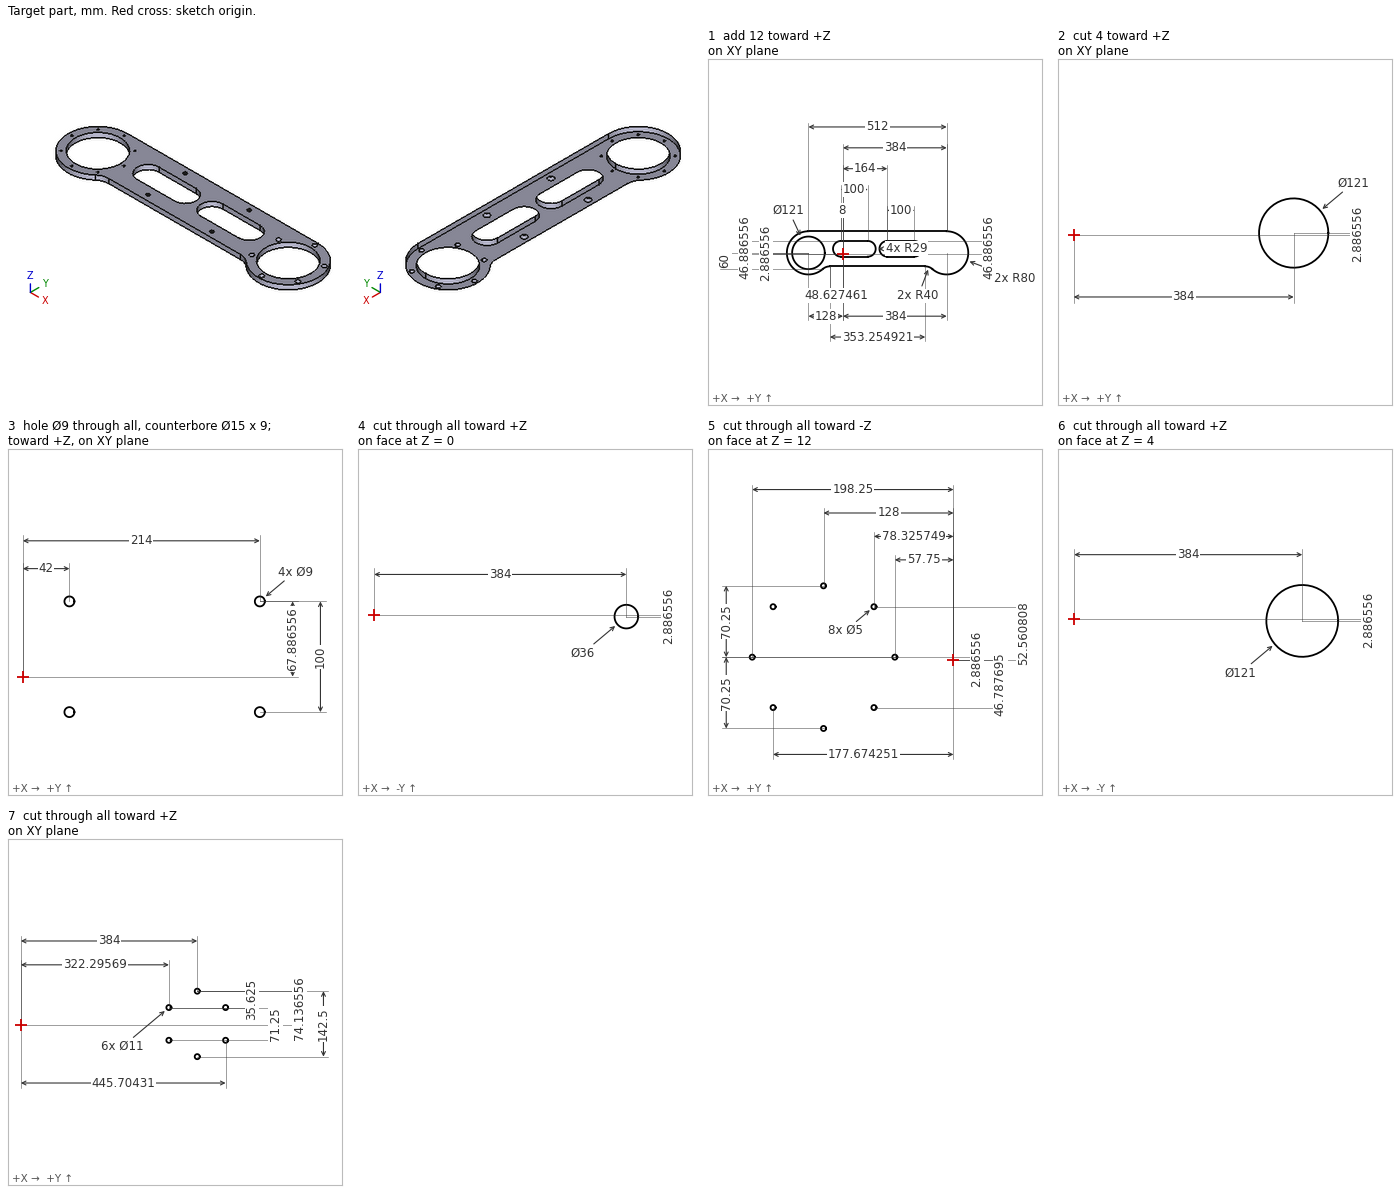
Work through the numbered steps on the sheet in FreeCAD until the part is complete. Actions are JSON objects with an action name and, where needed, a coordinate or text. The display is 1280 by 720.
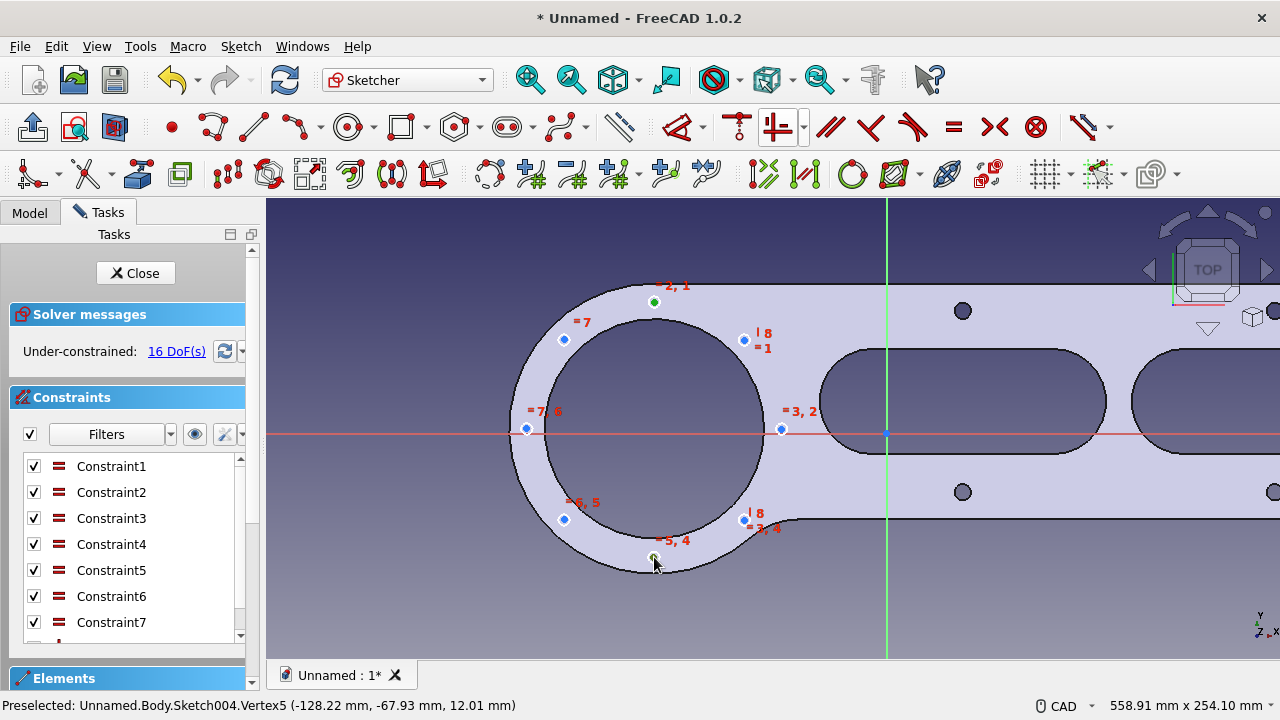
{"action": "left_click", "coordinate": [804, 128]}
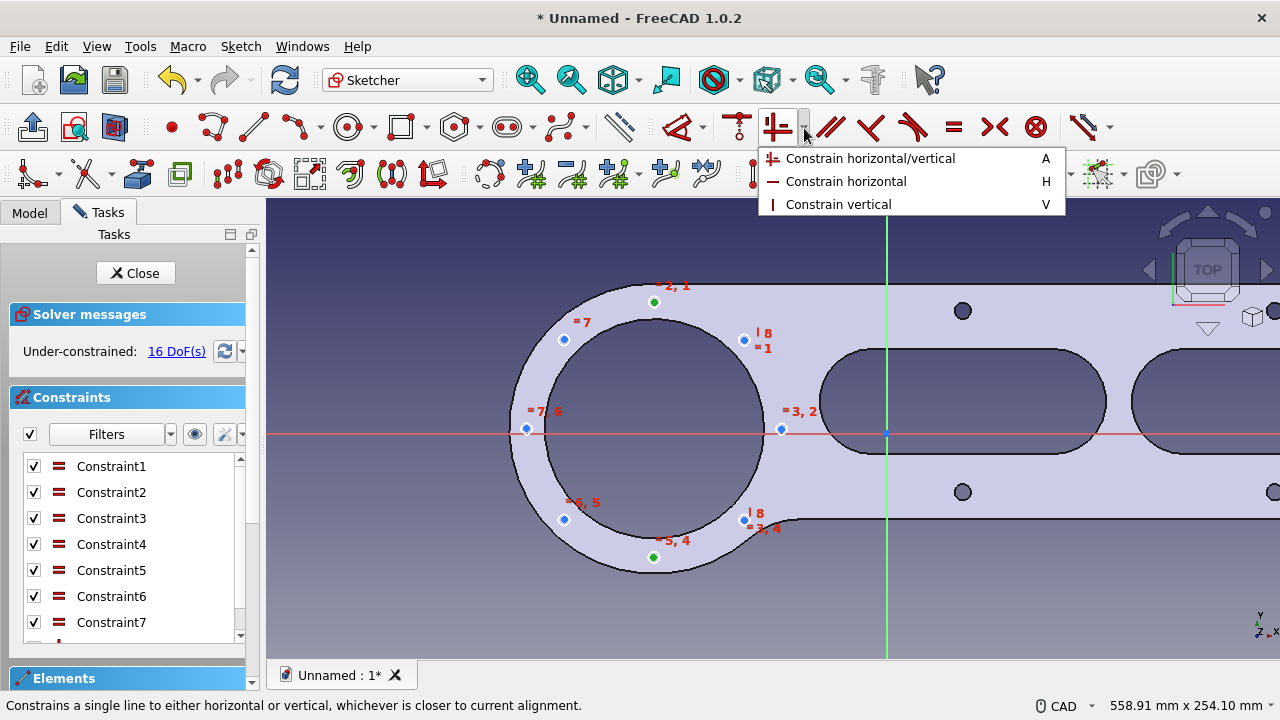
{"action": "left_click", "coordinate": [912, 204]}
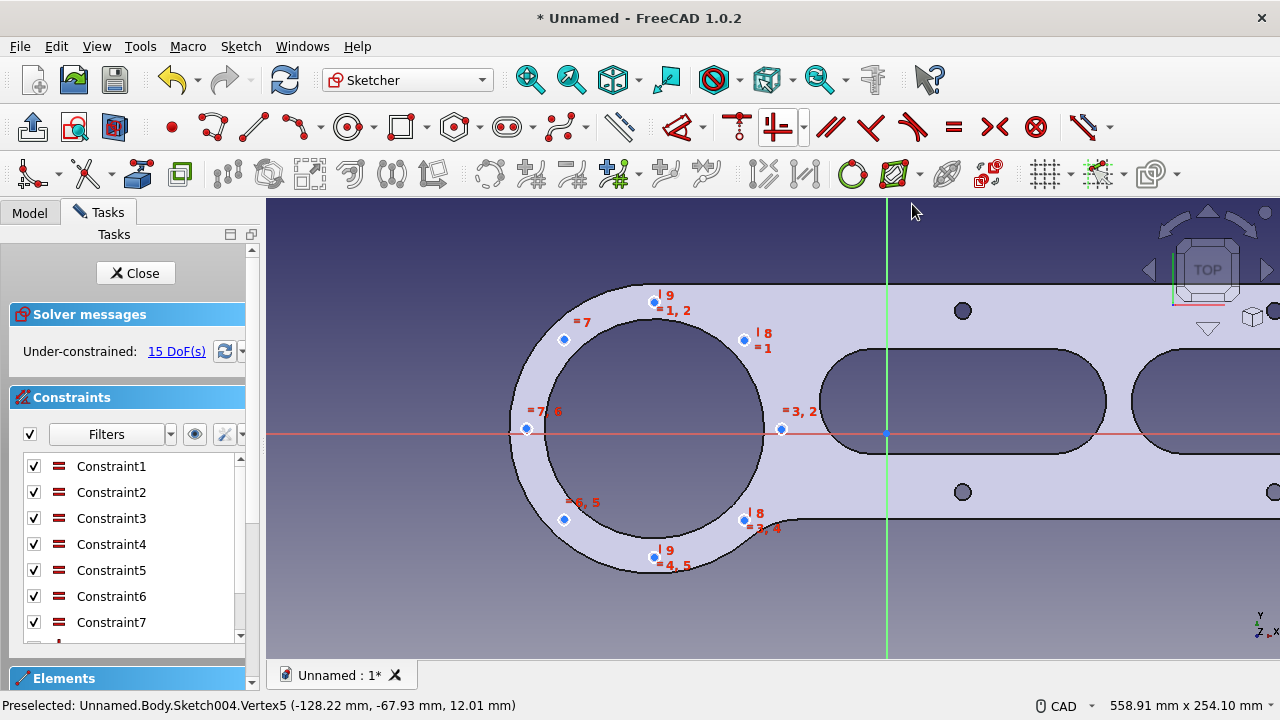
{"action": "left_click", "coordinate": [744, 520]}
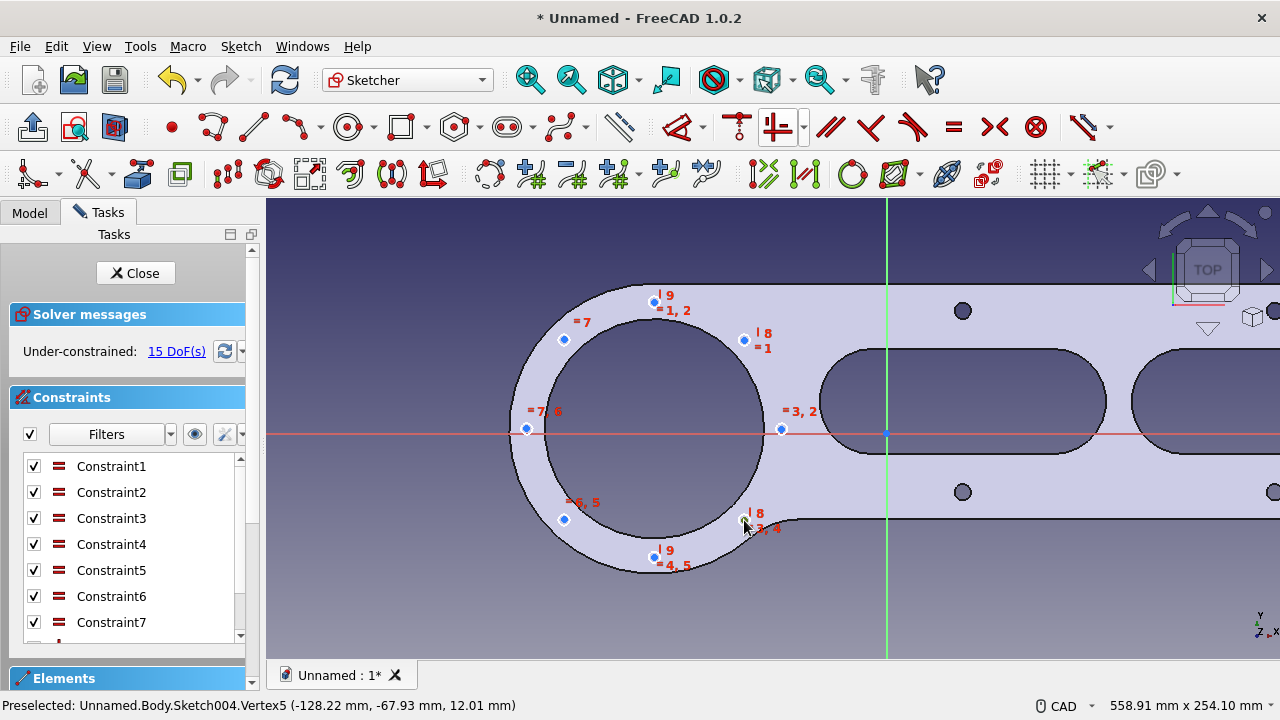
{"action": "left_click", "coordinate": [564, 520]}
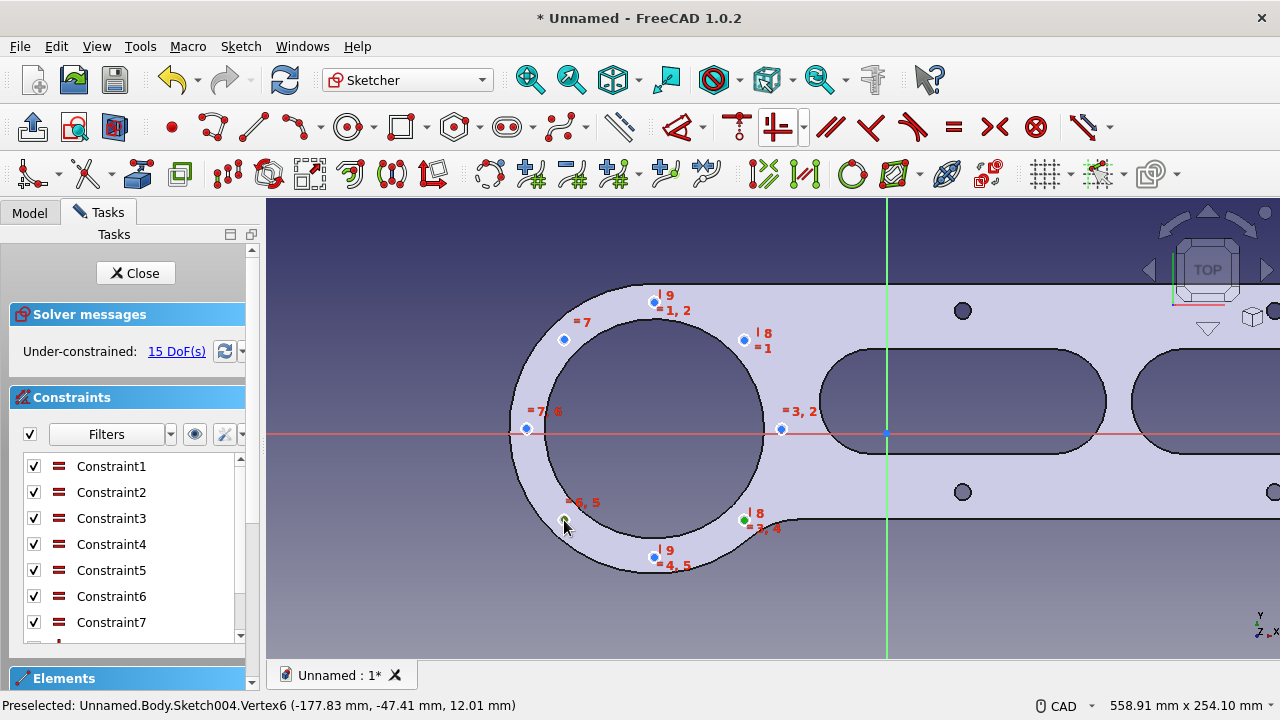
{"action": "left_click", "coordinate": [804, 128]}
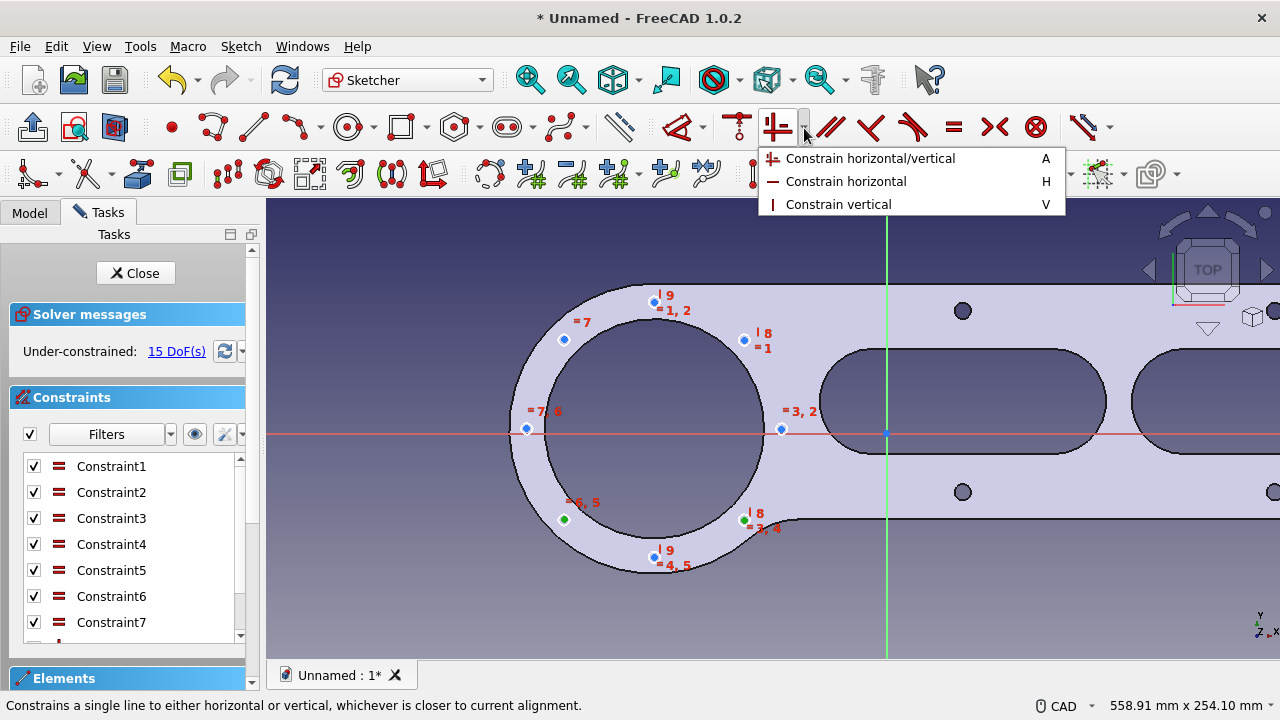
{"action": "left_click", "coordinate": [912, 182]}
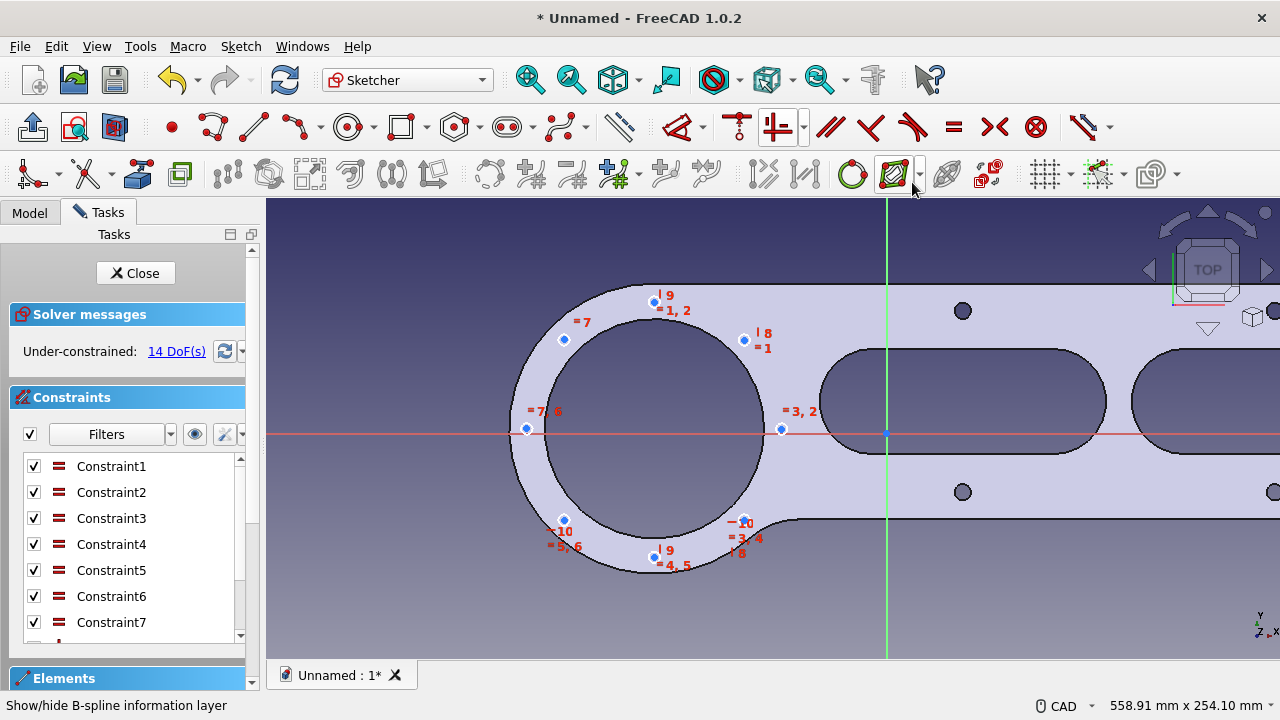
{"action": "left_click", "coordinate": [782, 429]}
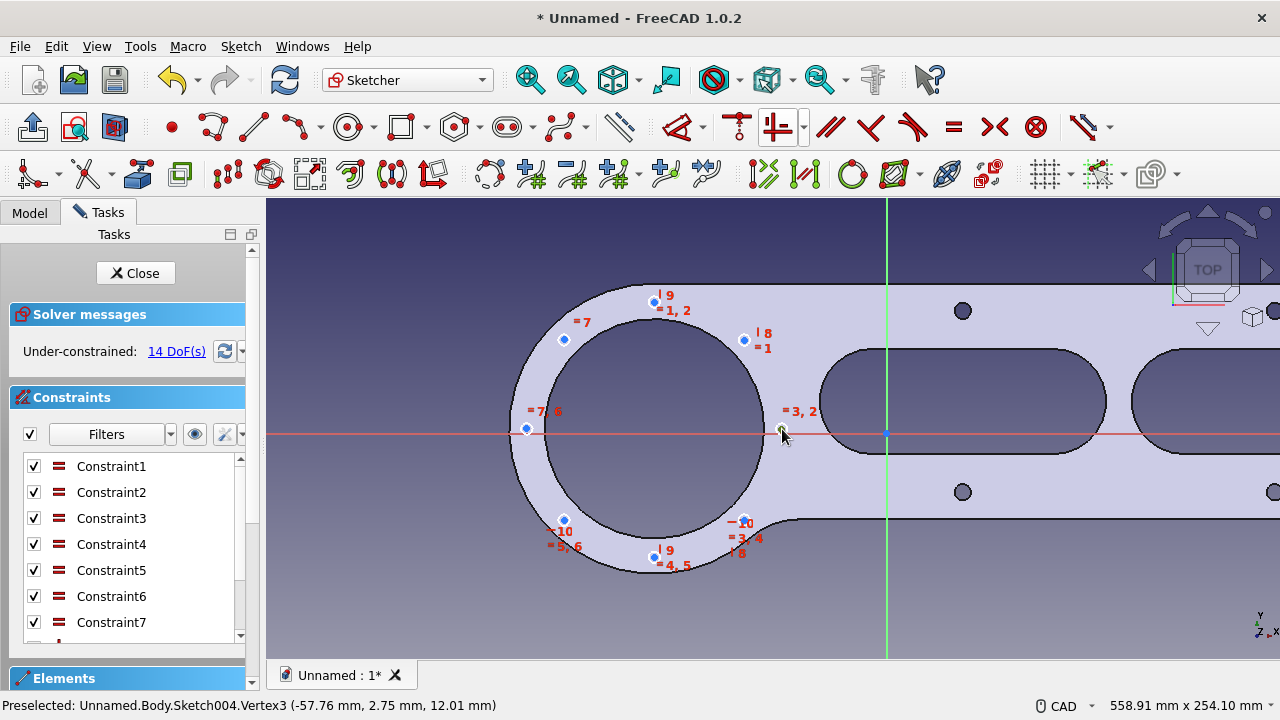
{"action": "left_click", "coordinate": [527, 429]}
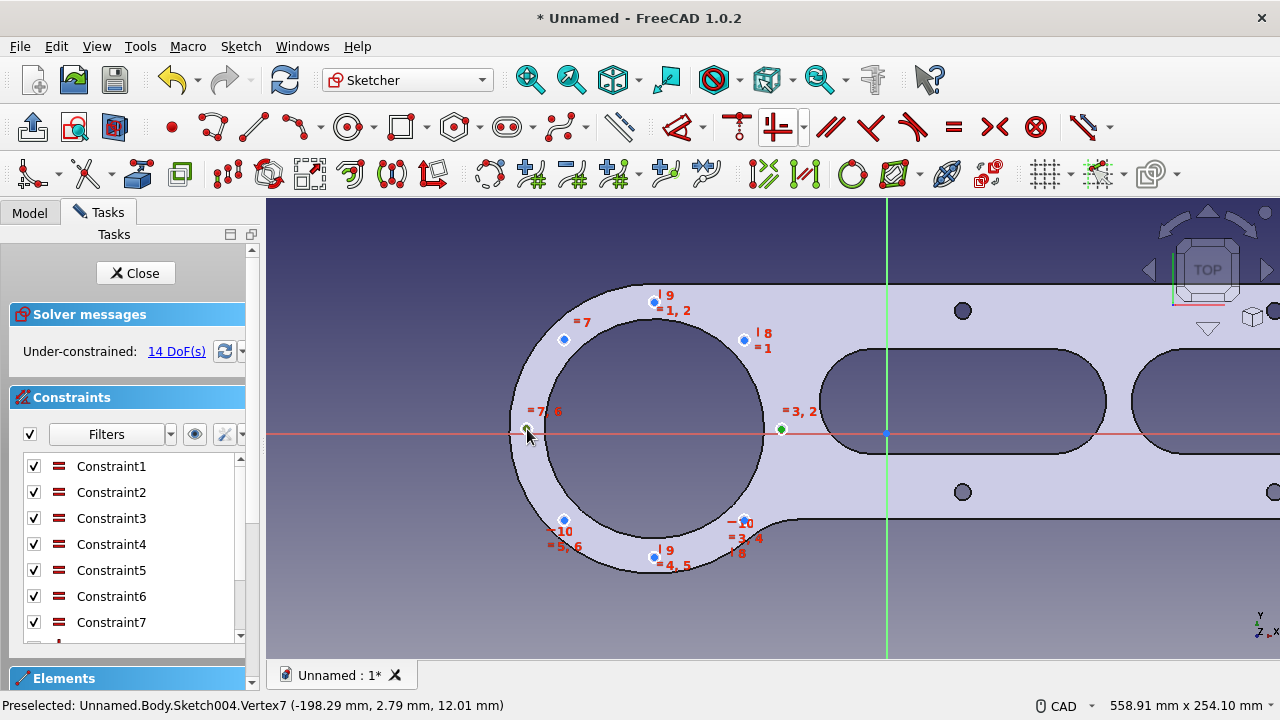
{"action": "left_click", "coordinate": [804, 128]}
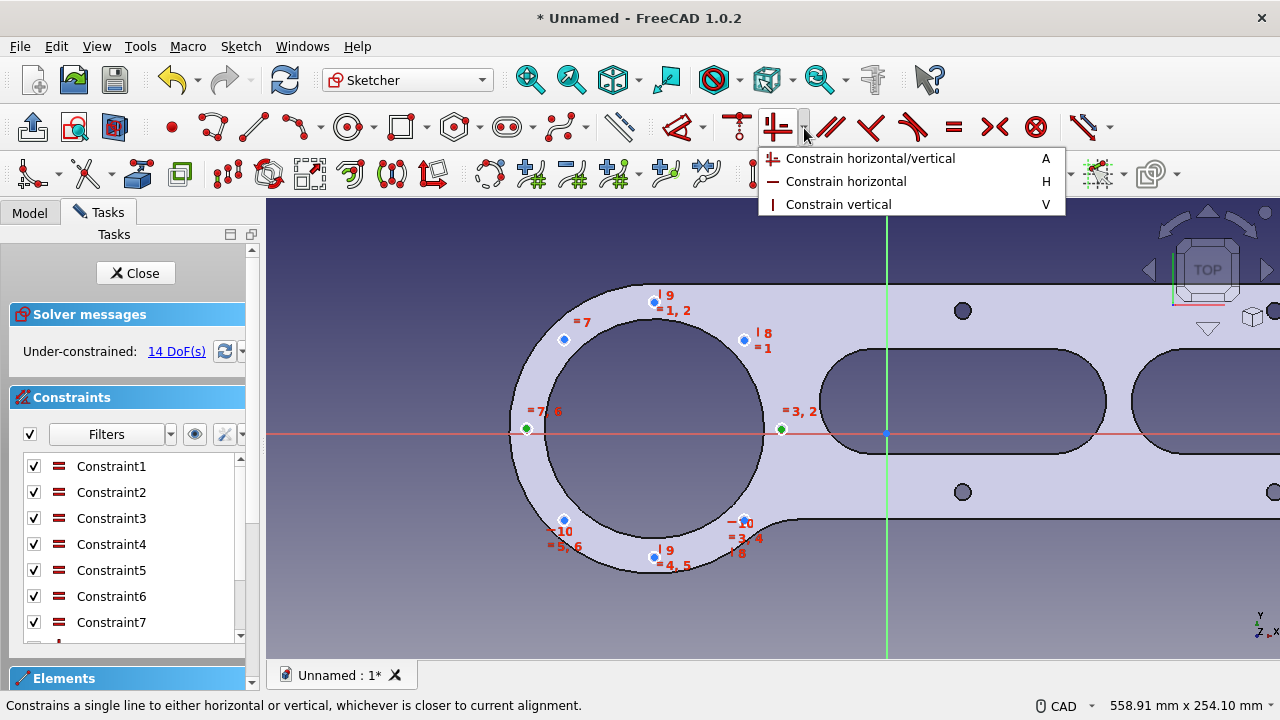
{"action": "left_click", "coordinate": [912, 182]}